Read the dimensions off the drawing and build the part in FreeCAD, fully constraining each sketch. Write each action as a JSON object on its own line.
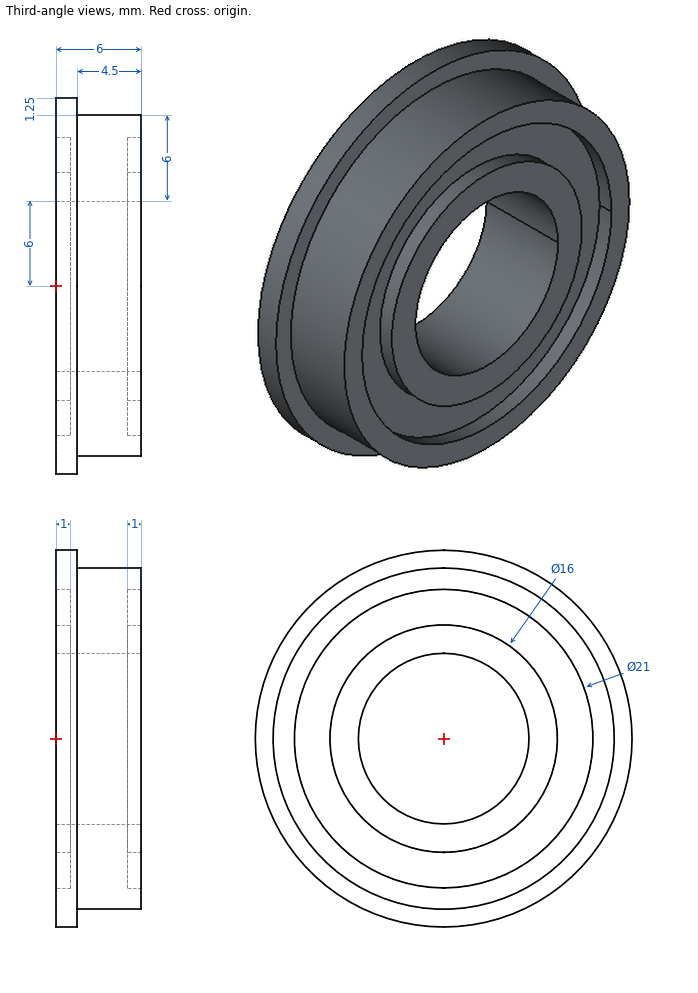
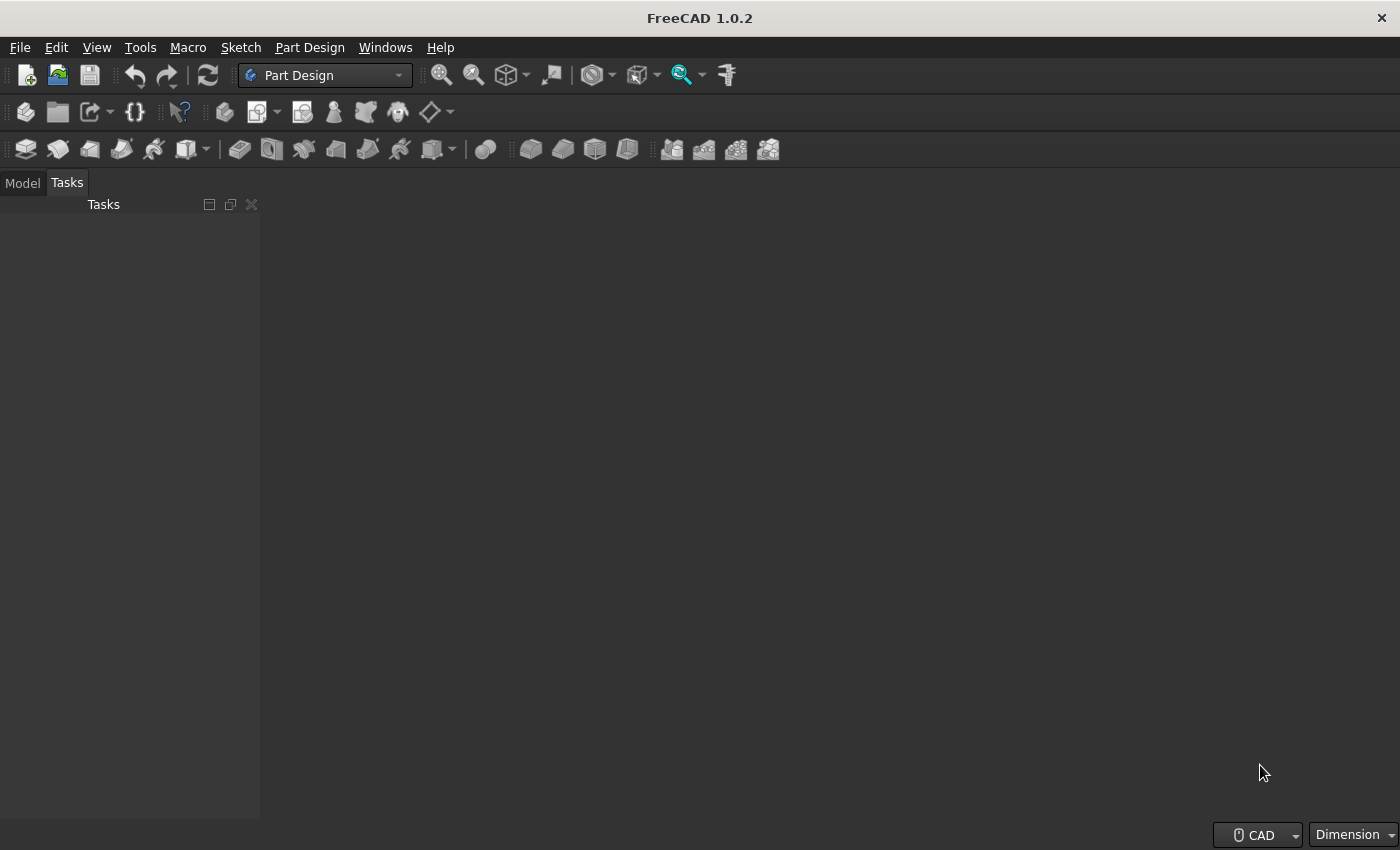
{"action": "left_click", "coordinate": [26, 76]}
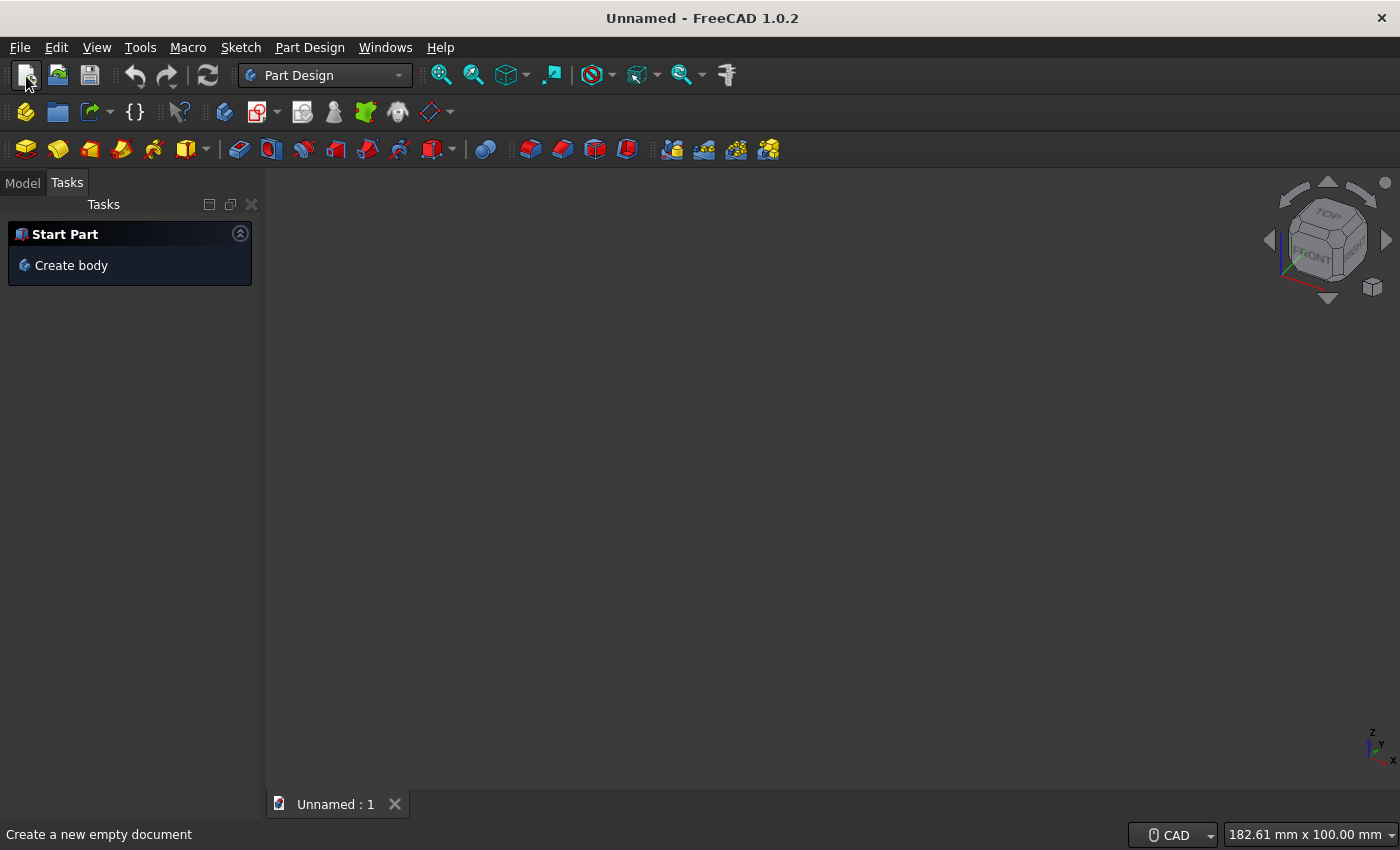
{"action": "left_click", "coordinate": [258, 112]}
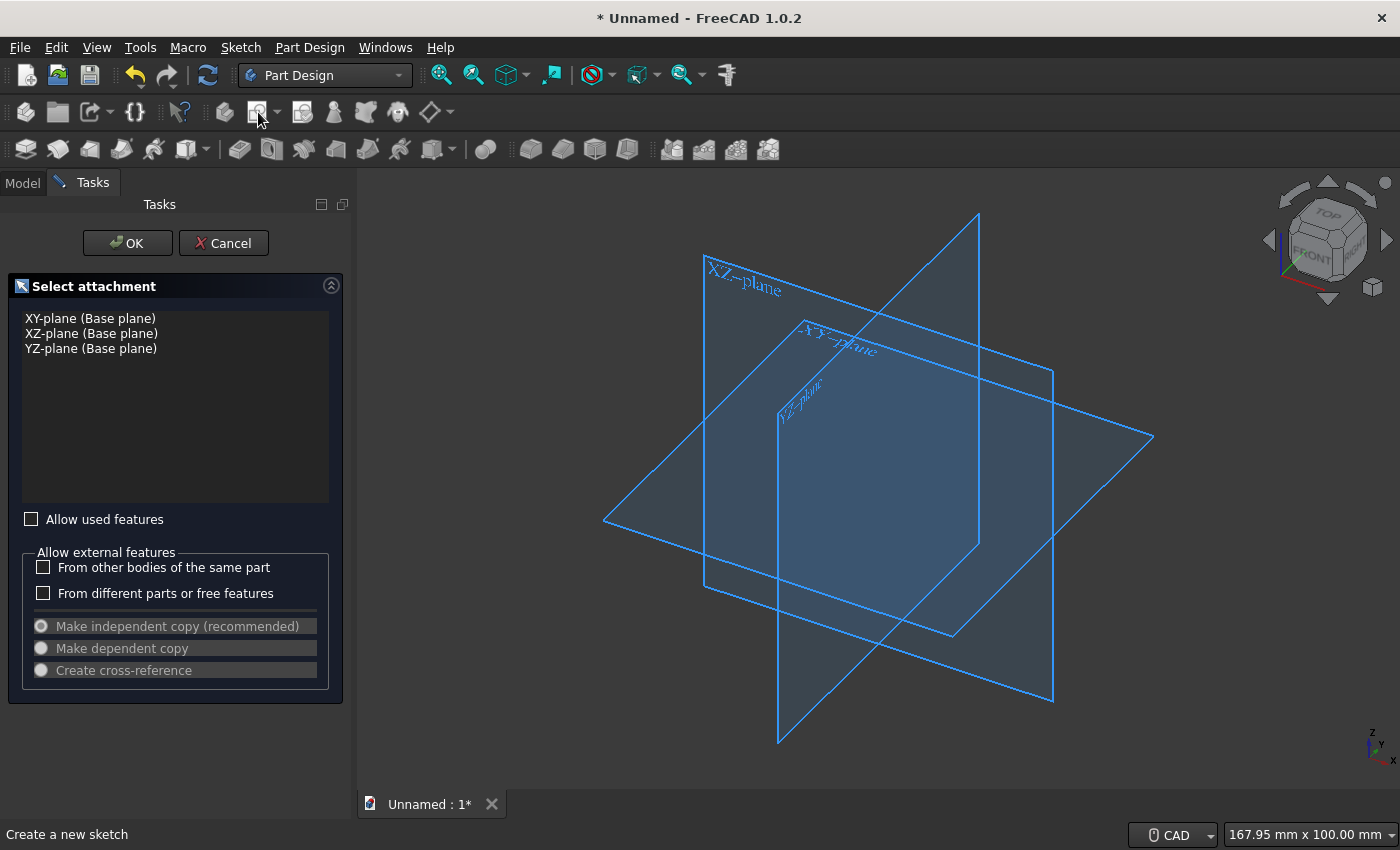
{"action": "left_click", "coordinate": [82, 318]}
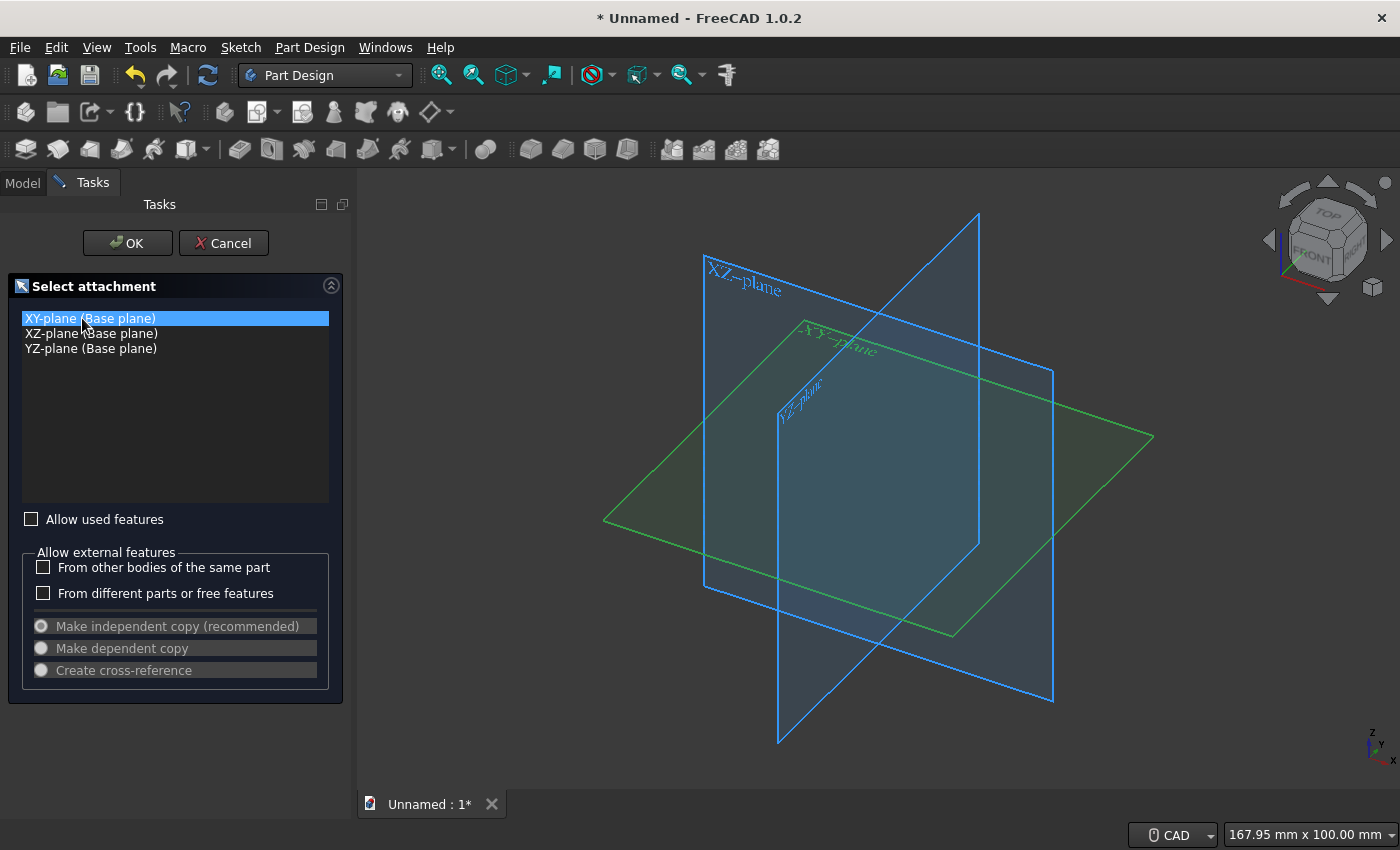
{"action": "left_click", "coordinate": [128, 243]}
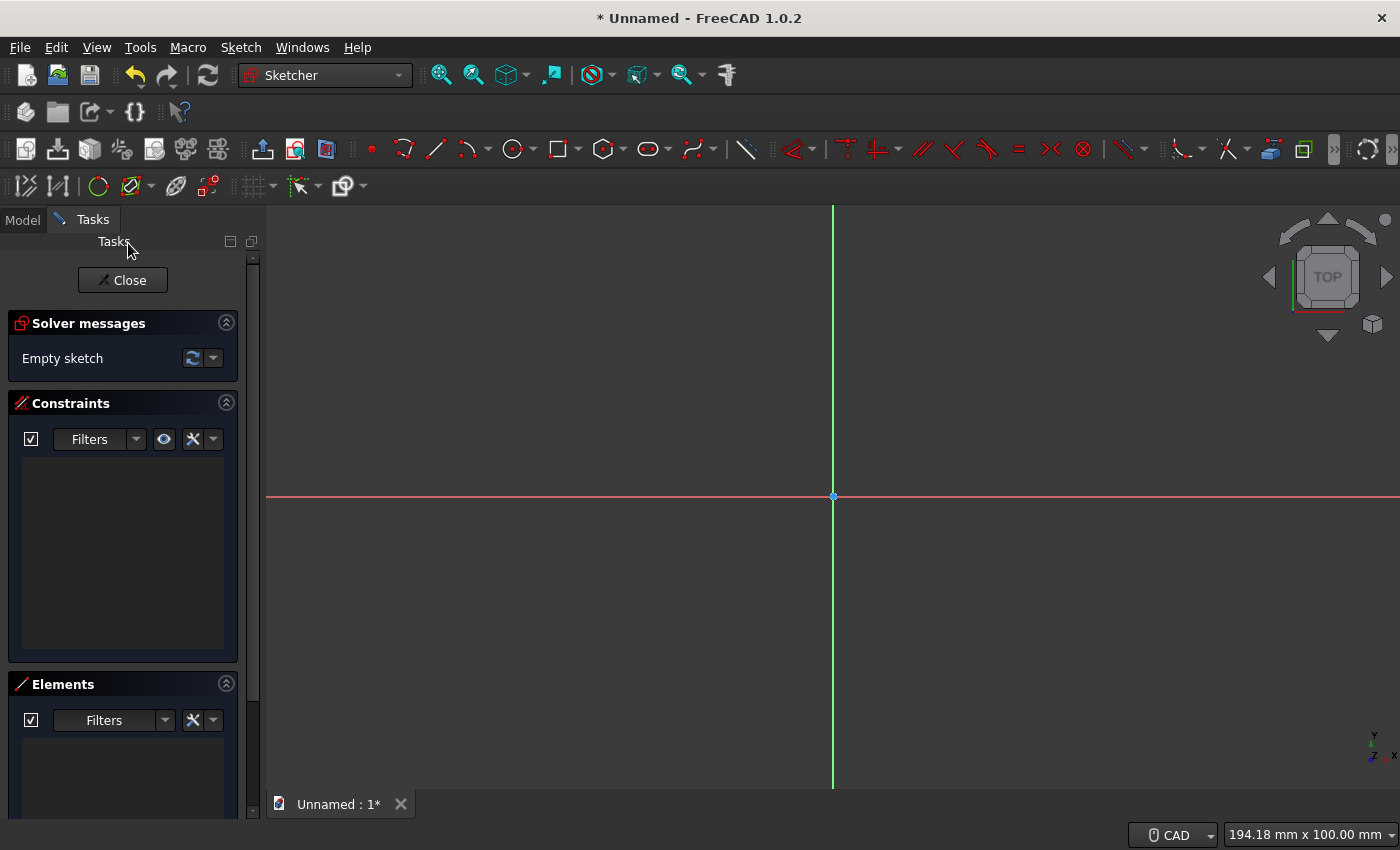
{"action": "scroll", "coordinate": [872, 449], "scroll_direction": "up", "scroll_amount": 8}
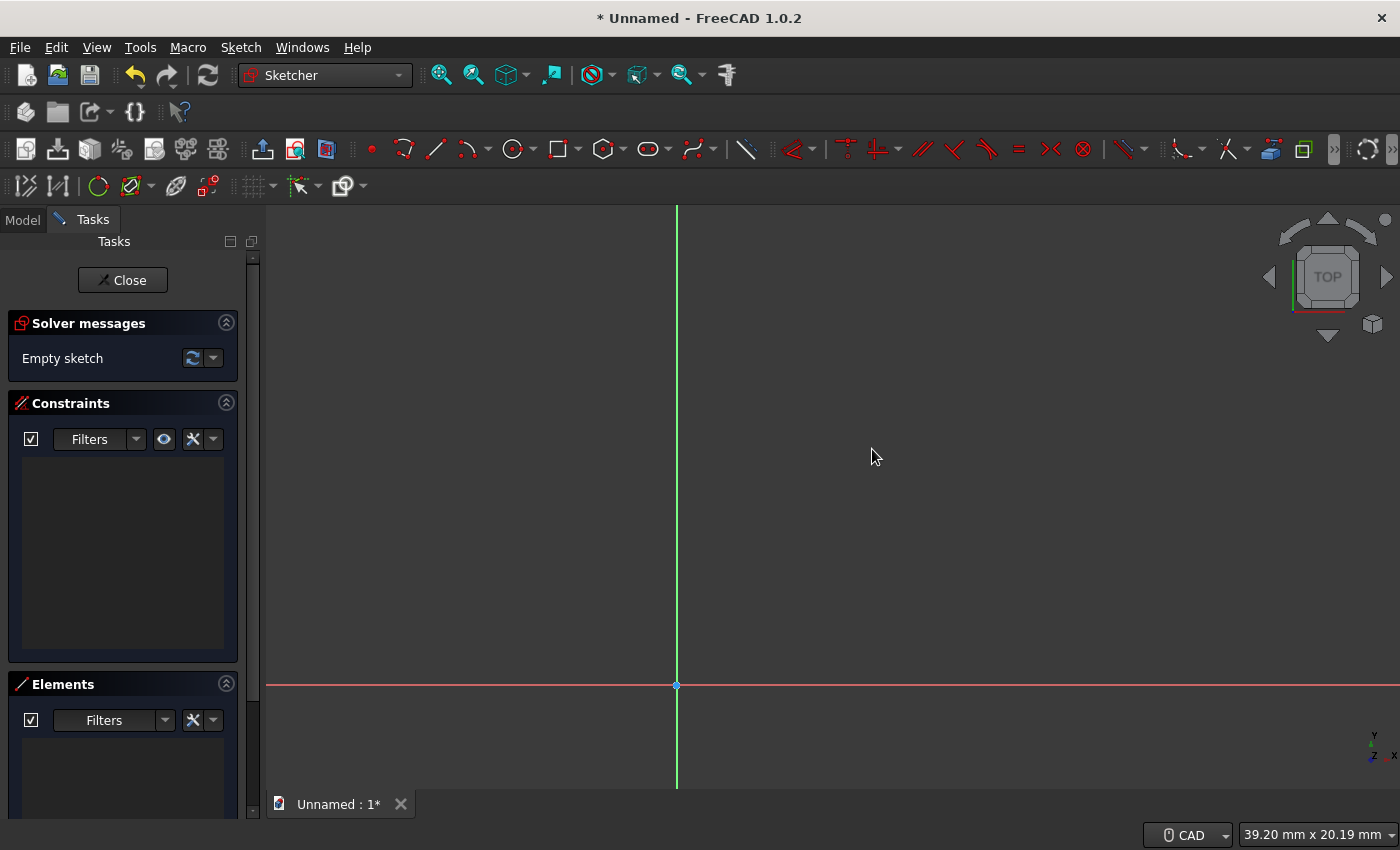
{"action": "left_click", "coordinate": [404, 150]}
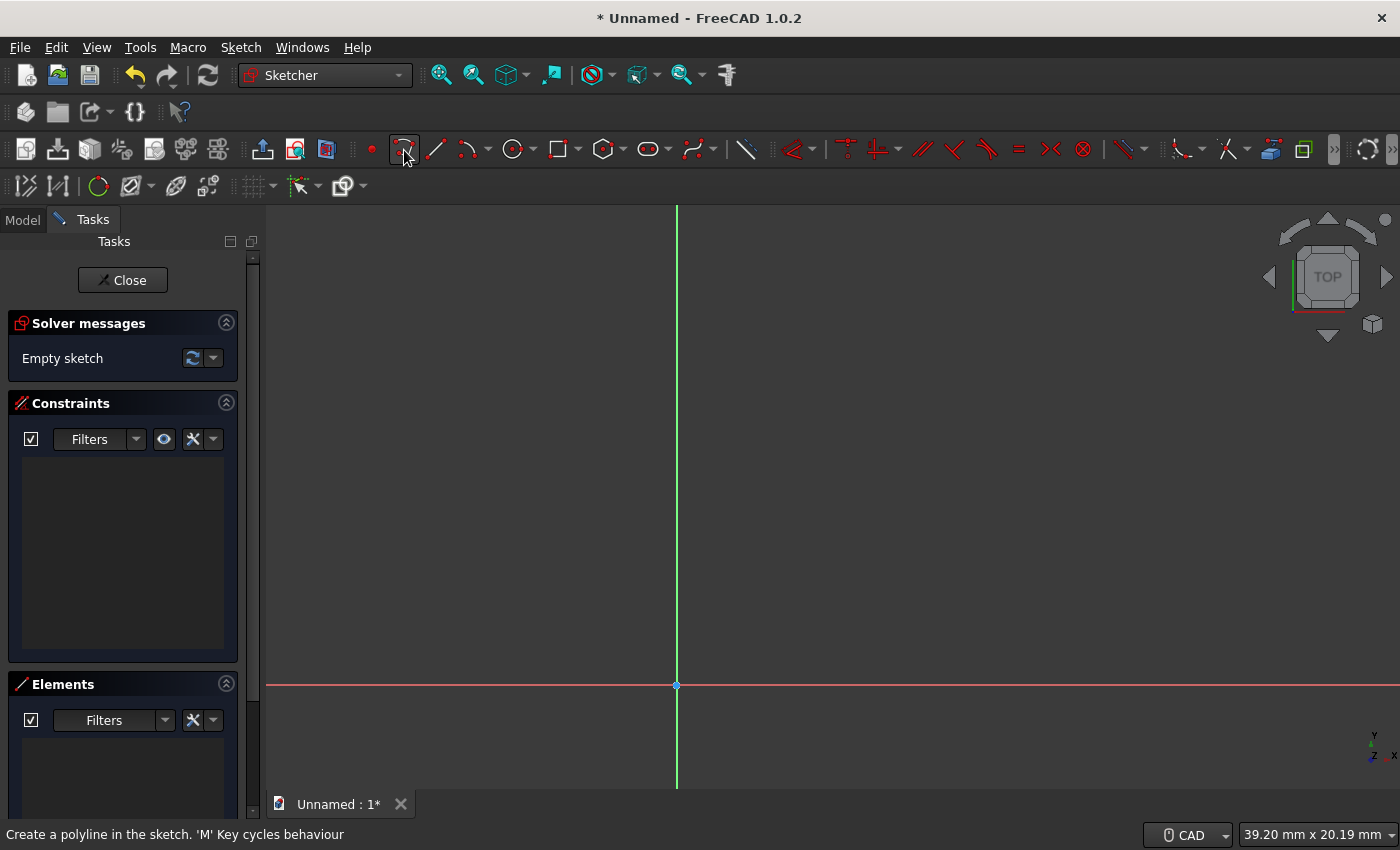
{"action": "left_click", "coordinate": [677, 512]}
{"action": "left_click", "coordinate": [850, 512]}
{"action": "left_click", "coordinate": [850, 338]}
{"action": "left_click", "coordinate": [720, 338]}
{"action": "left_click", "coordinate": [720, 302]}
{"action": "left_click", "coordinate": [686, 302]}
{"action": "left_click", "coordinate": [677, 513]}
{"action": "key", "text": "Escape"}
{"action": "key", "text": "Escape"}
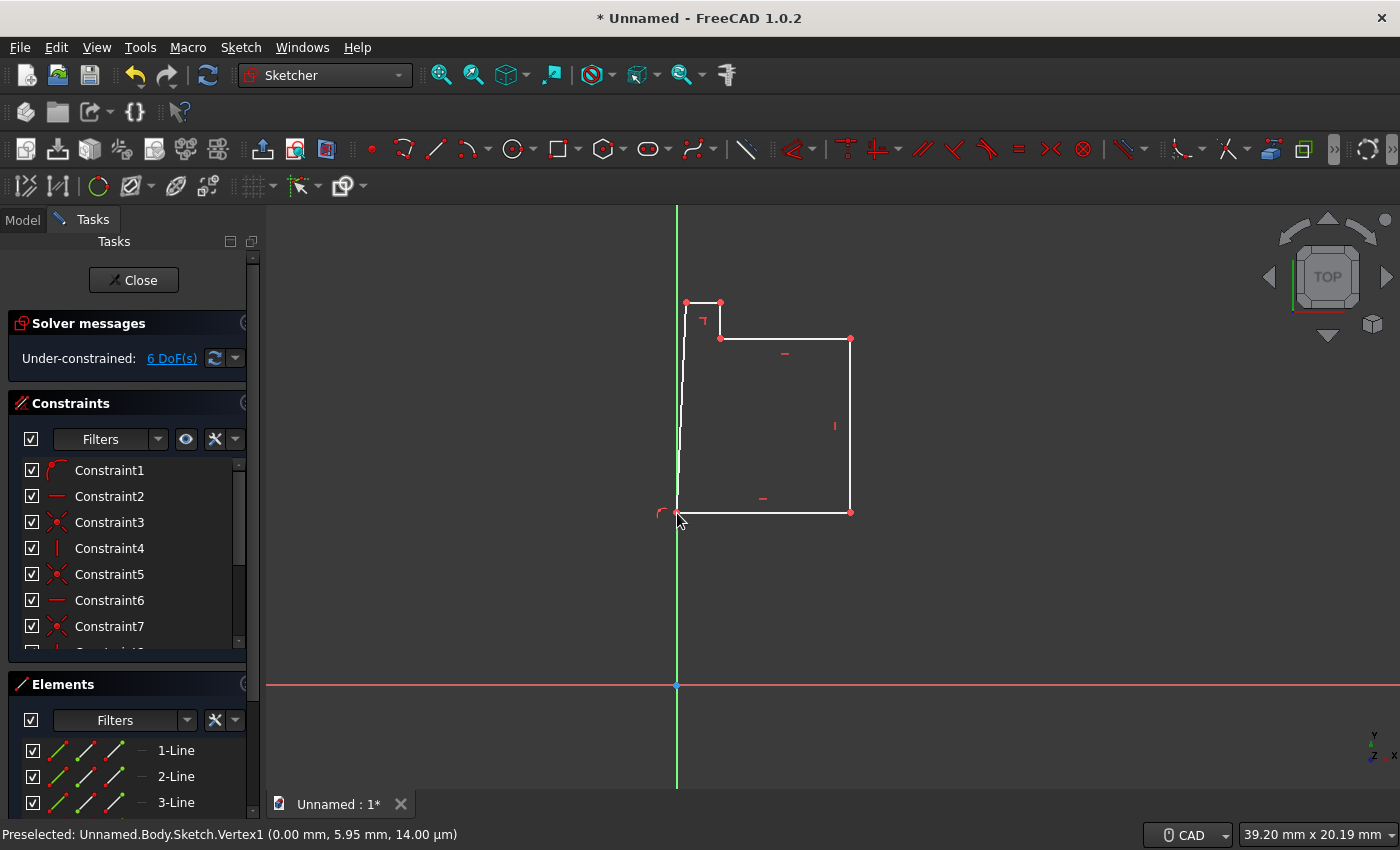
{"action": "left_click", "coordinate": [680, 450]}